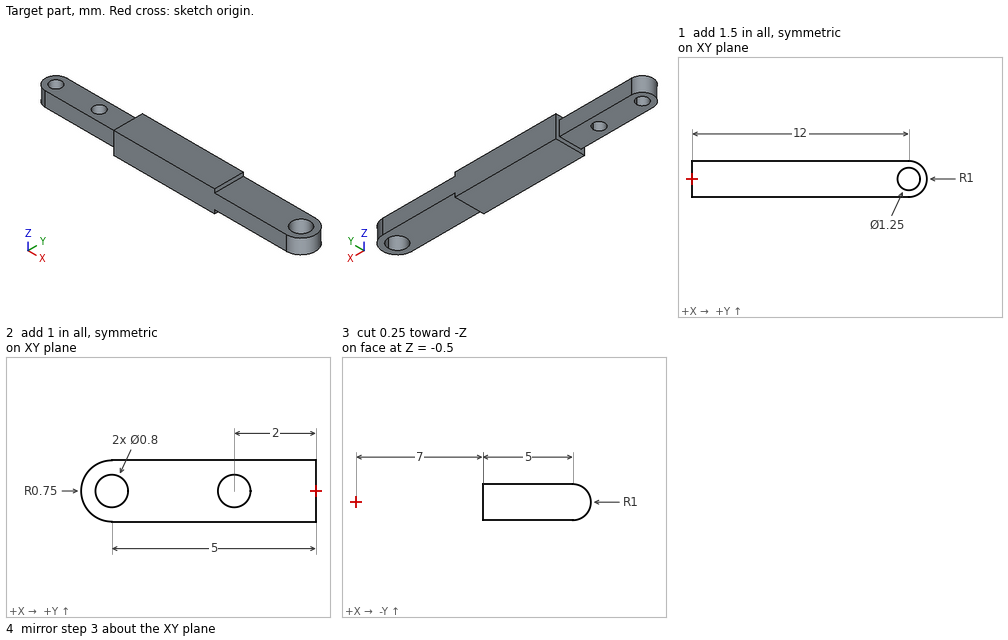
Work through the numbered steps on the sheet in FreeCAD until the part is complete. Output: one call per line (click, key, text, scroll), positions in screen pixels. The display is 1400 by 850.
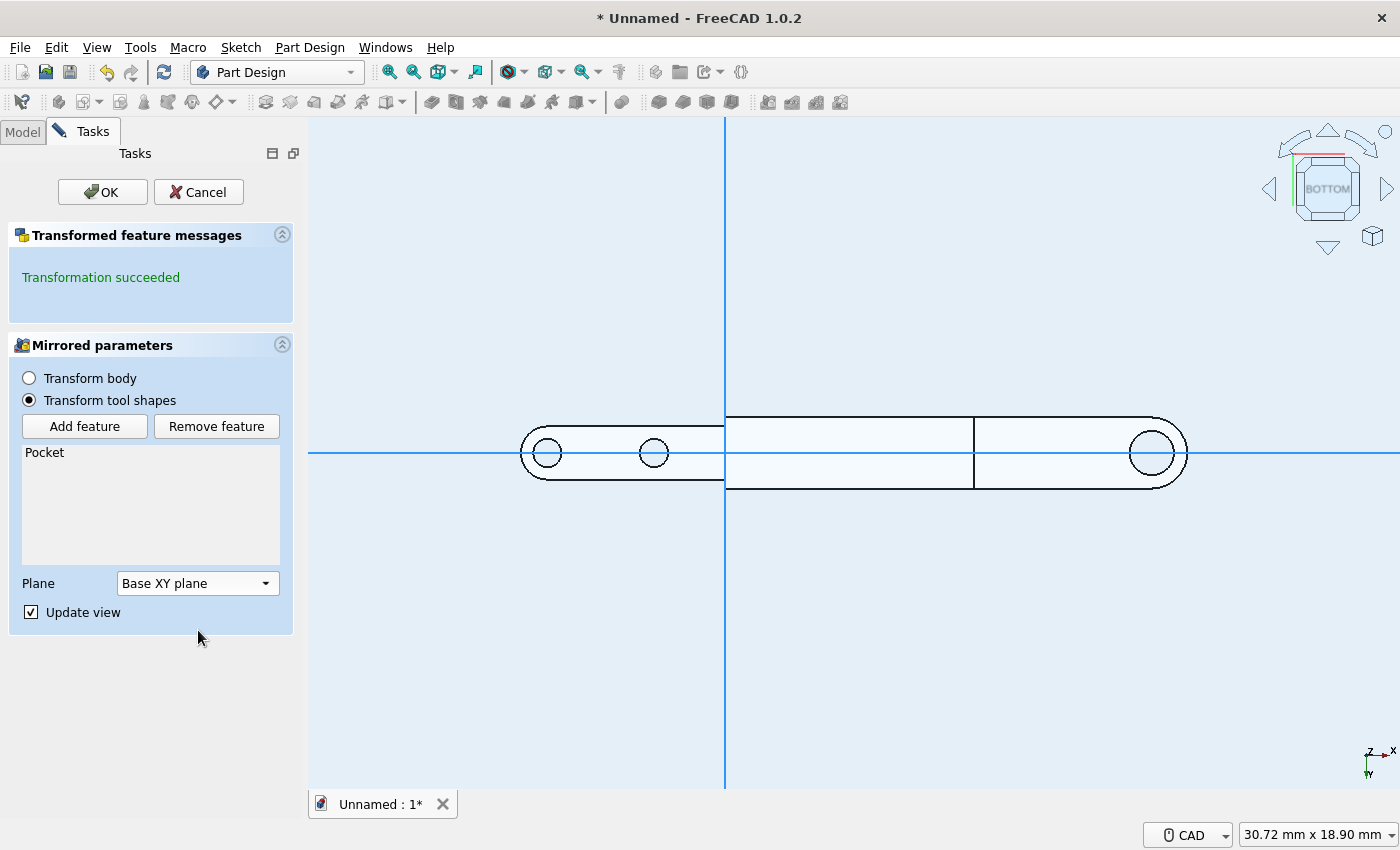
click(103, 192)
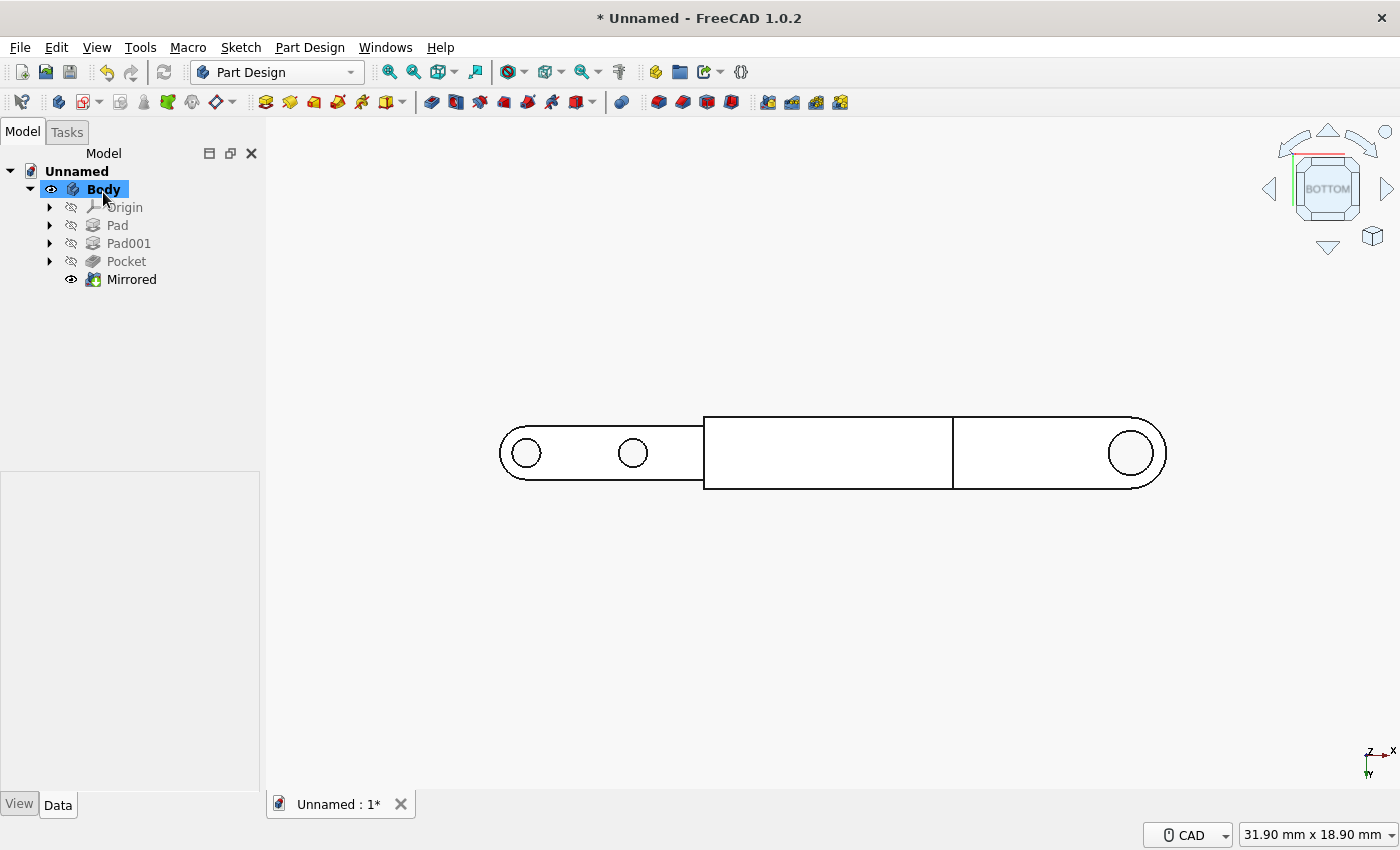
key(0)